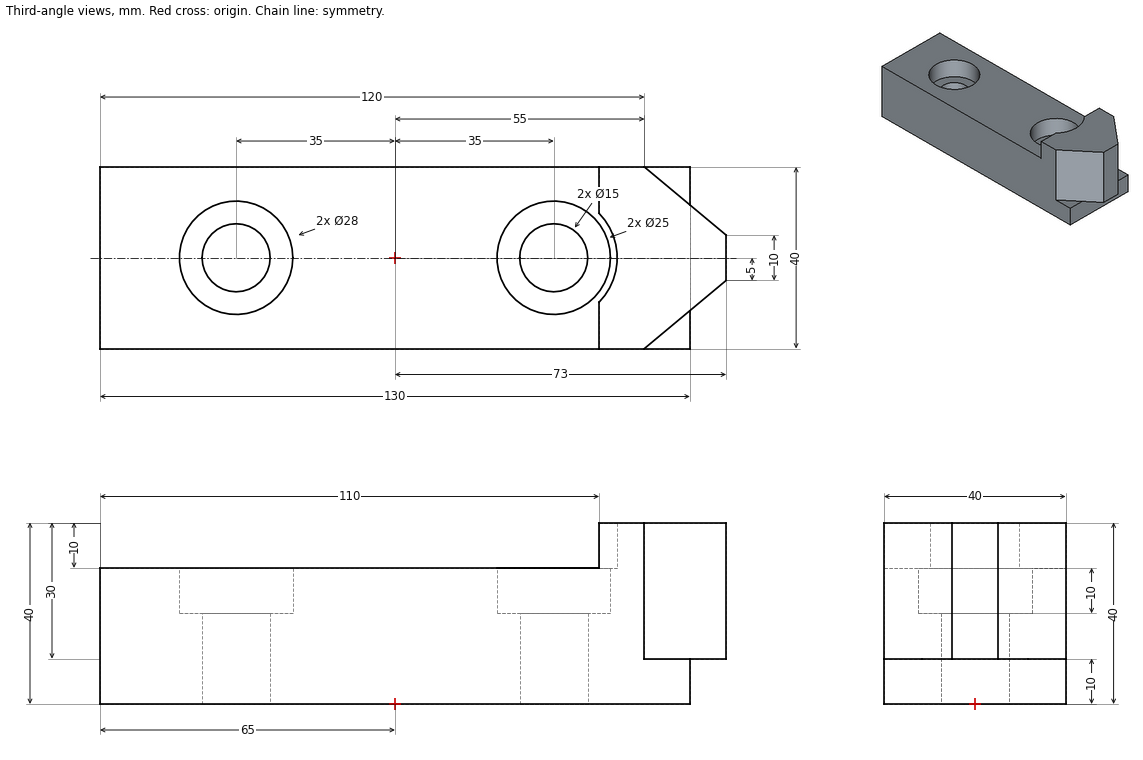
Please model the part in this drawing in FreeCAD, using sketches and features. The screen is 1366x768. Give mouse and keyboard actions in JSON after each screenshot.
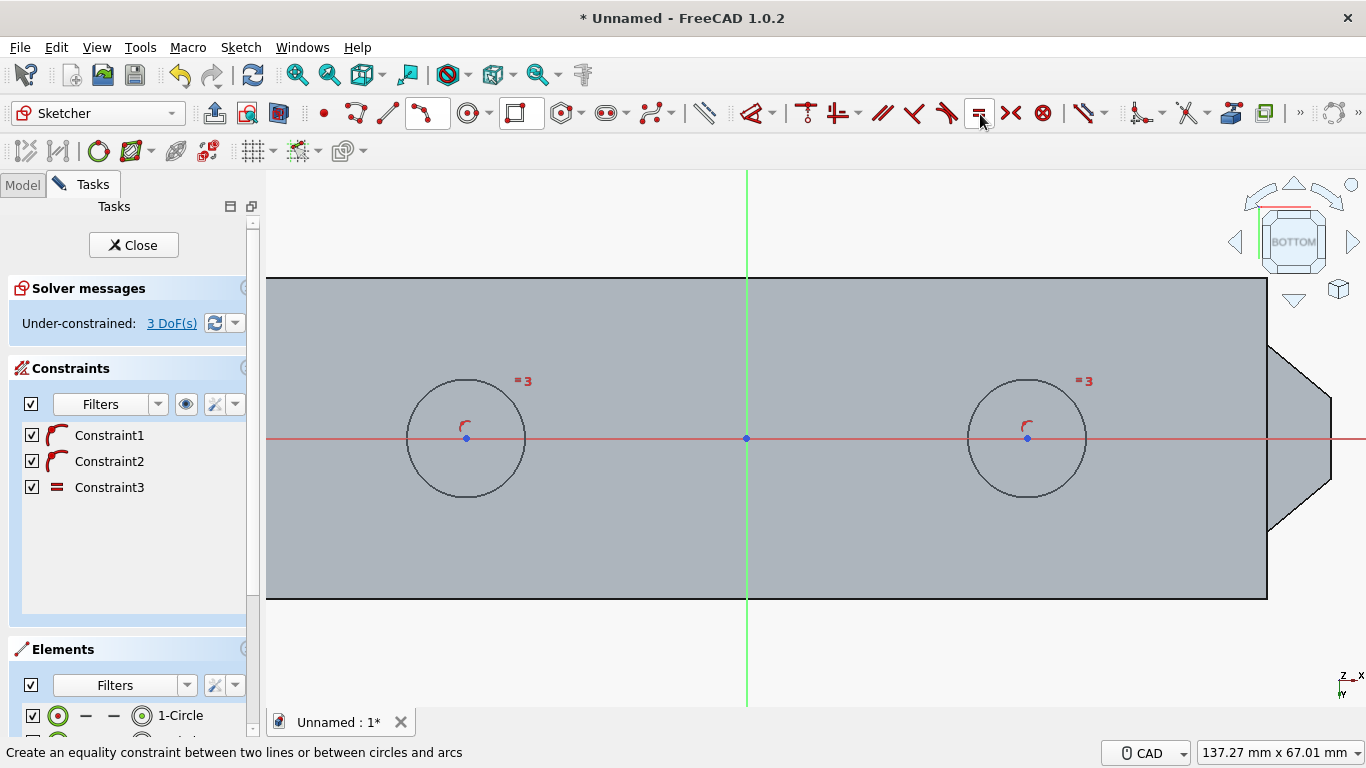
{"action": "left_click", "coordinate": [752, 114]}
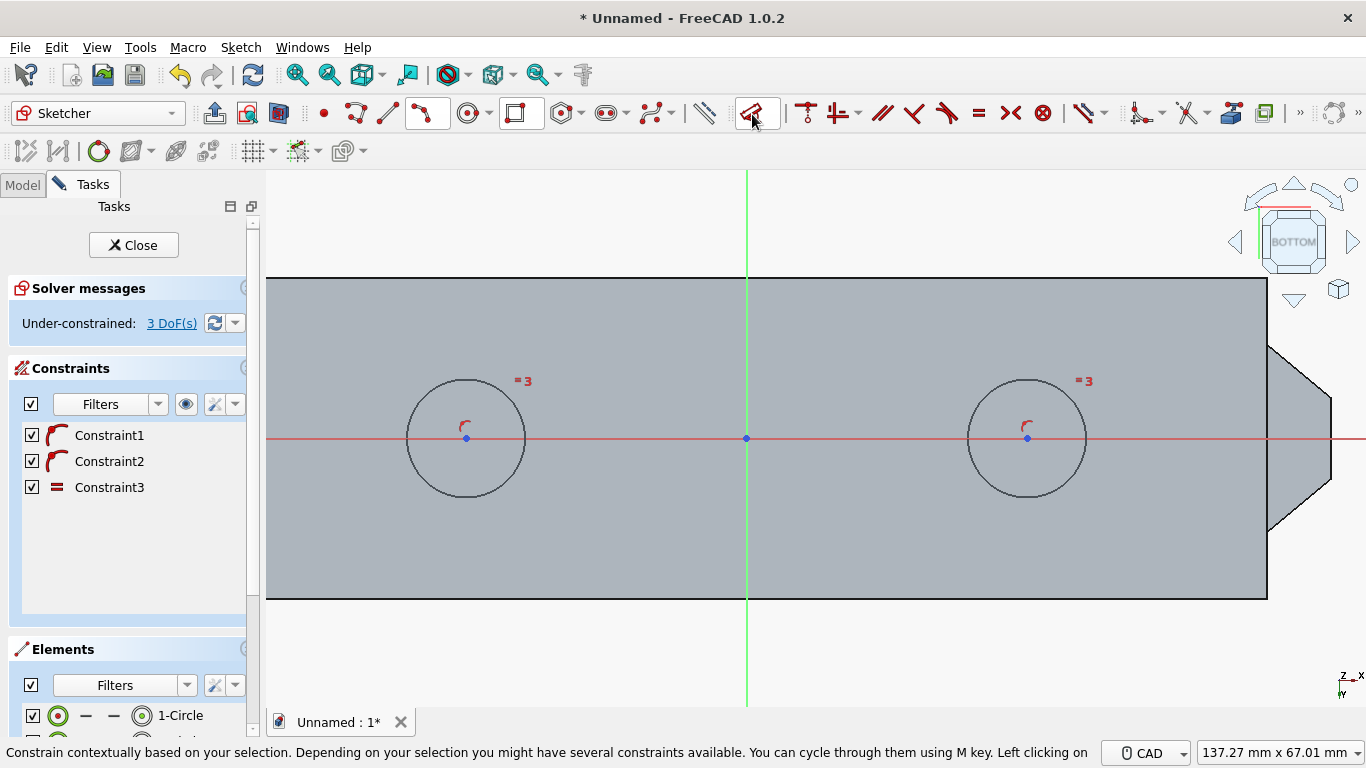
{"action": "left_click", "coordinate": [1069, 397]}
{"action": "left_click", "coordinate": [1092, 375]}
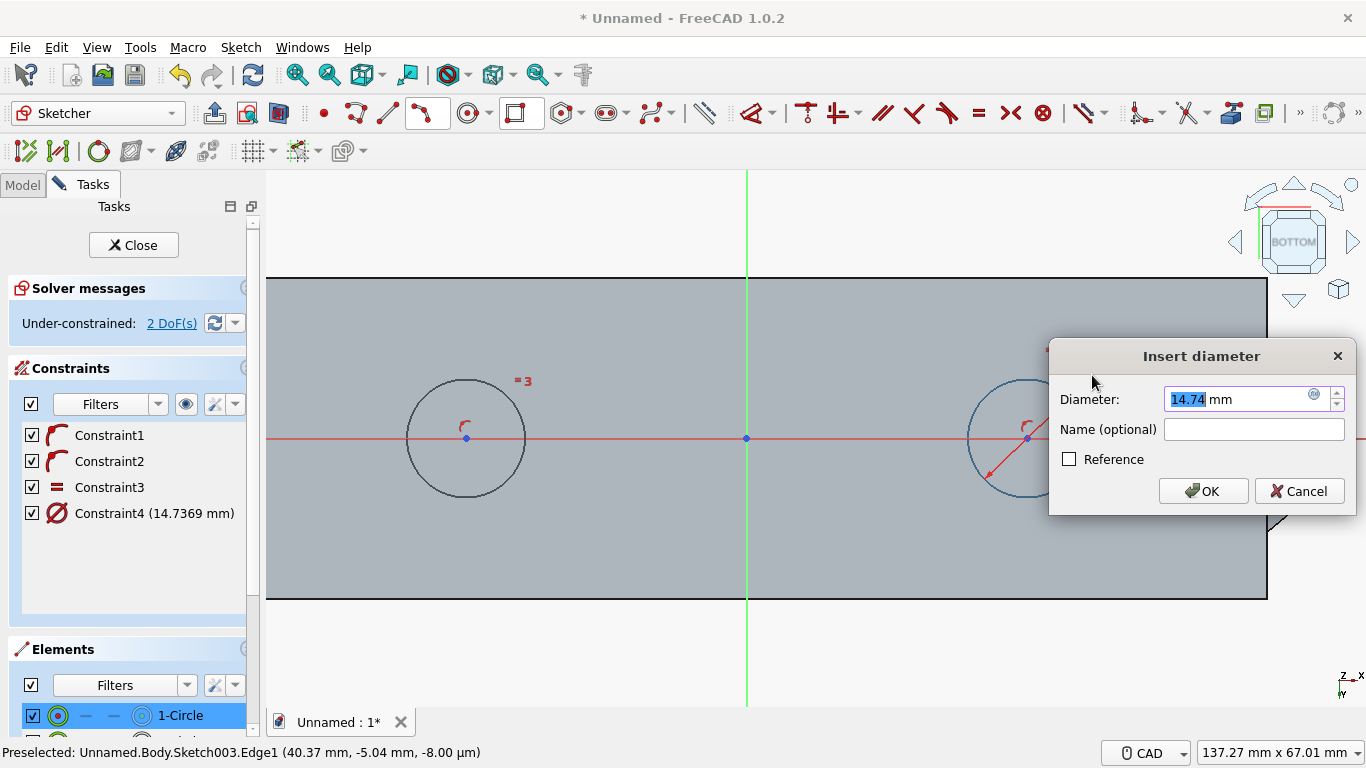
{"action": "type", "text": "15"}
{"action": "key", "text": "Return"}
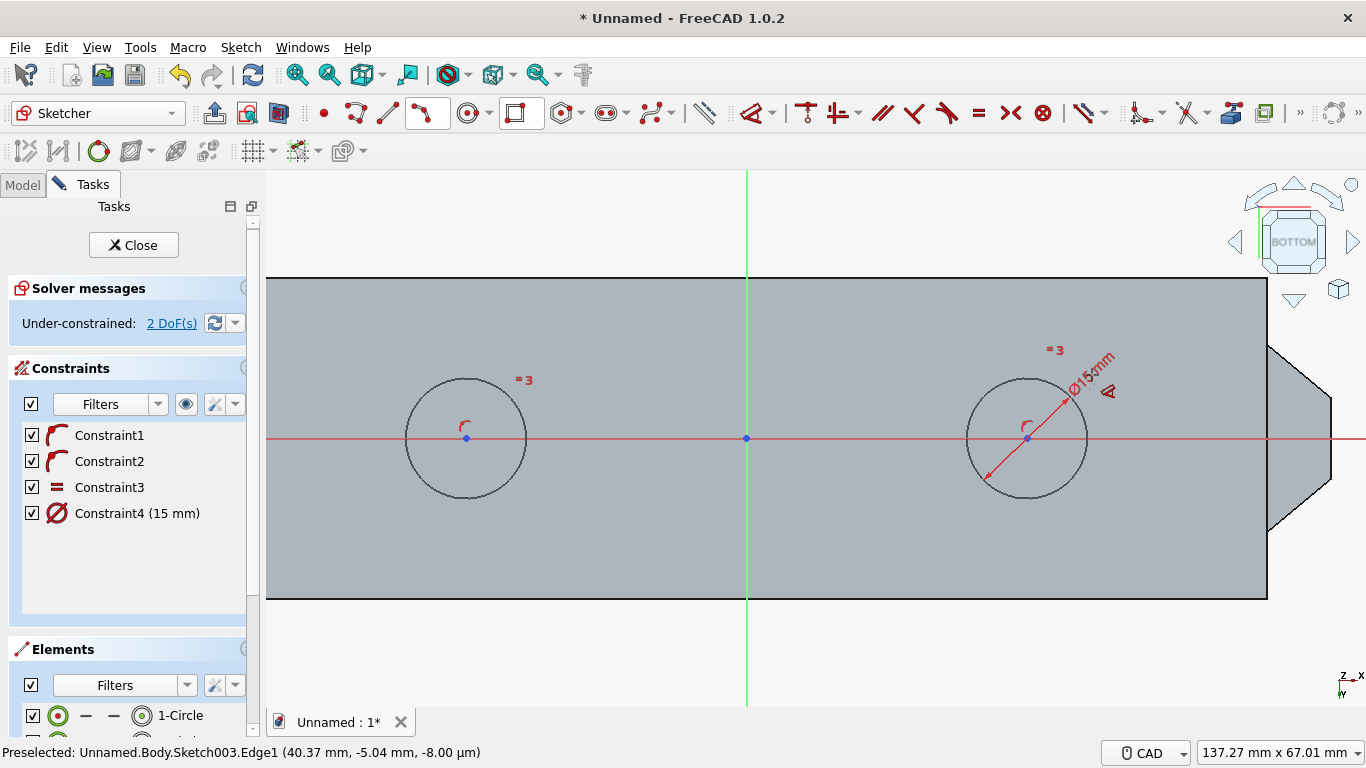
{"action": "left_click", "coordinate": [1027, 438]}
{"action": "left_click", "coordinate": [887, 472]}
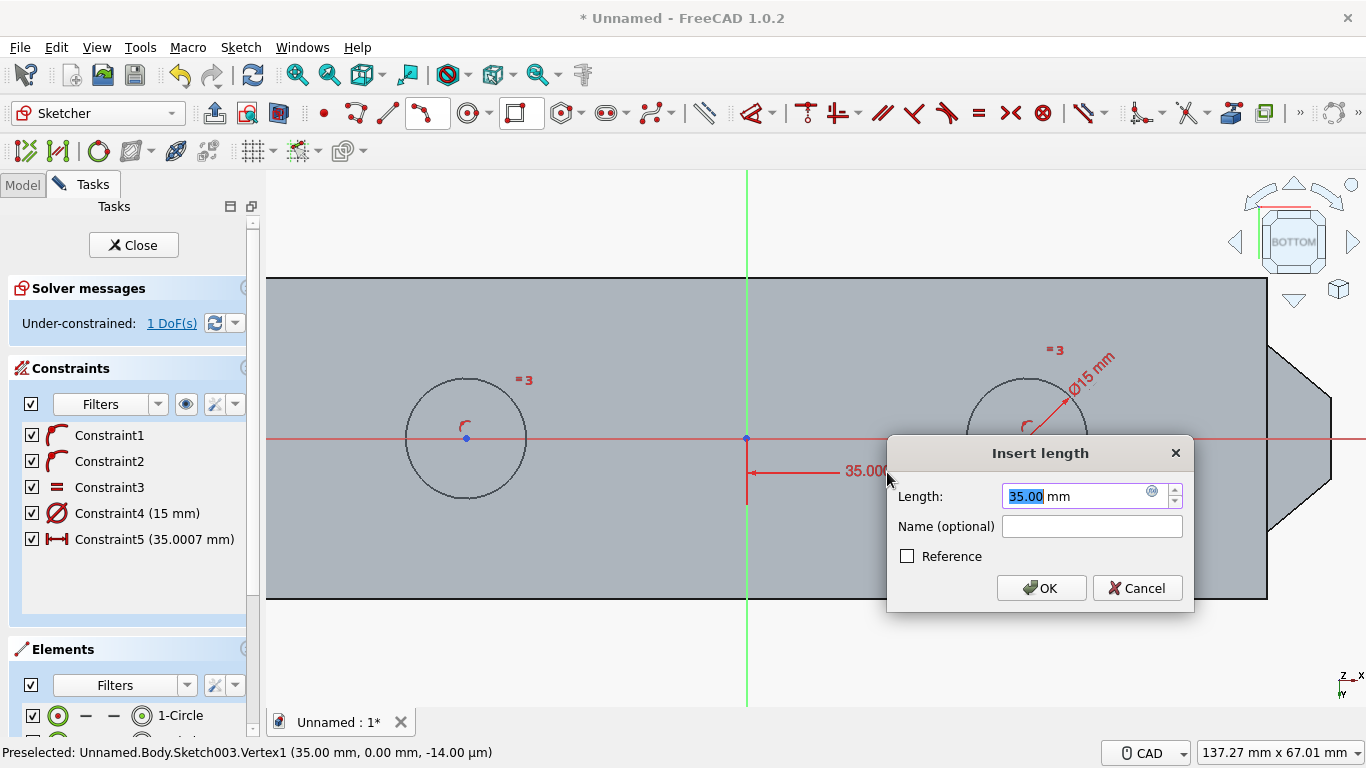
{"action": "type", "text": "35"}
{"action": "key", "text": "Return"}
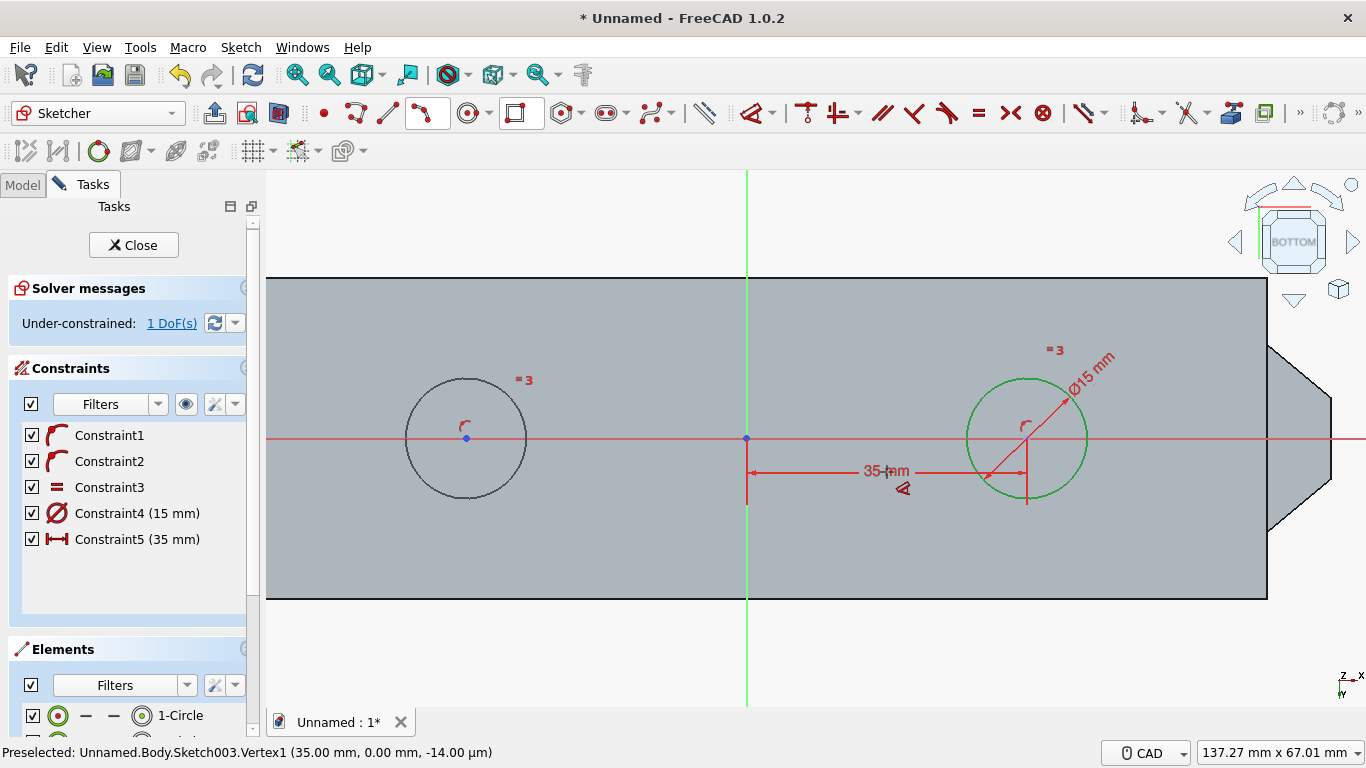
{"action": "left_click", "coordinate": [466, 438]}
{"action": "left_click", "coordinate": [606, 472]}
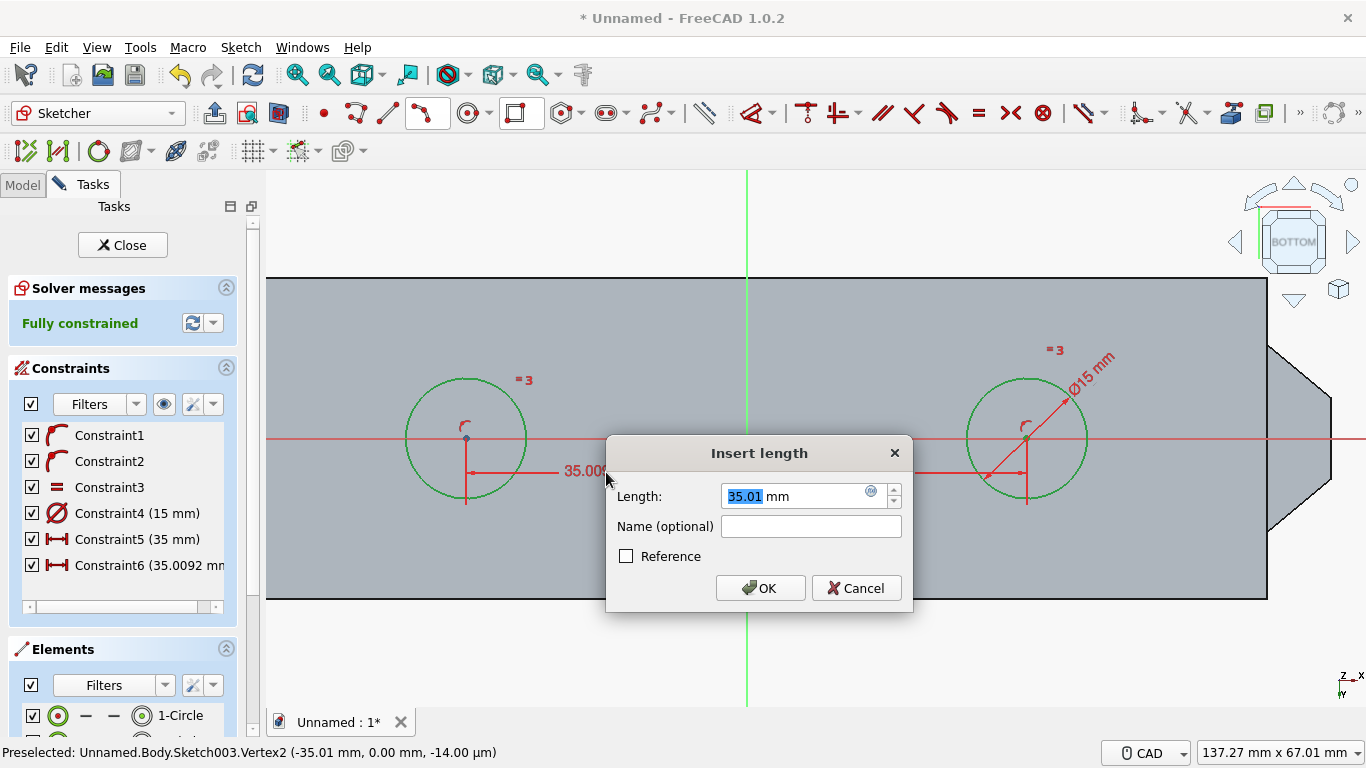
{"action": "type", "text": "35"}
{"action": "key", "text": "Return"}
{"action": "key", "text": "Escape"}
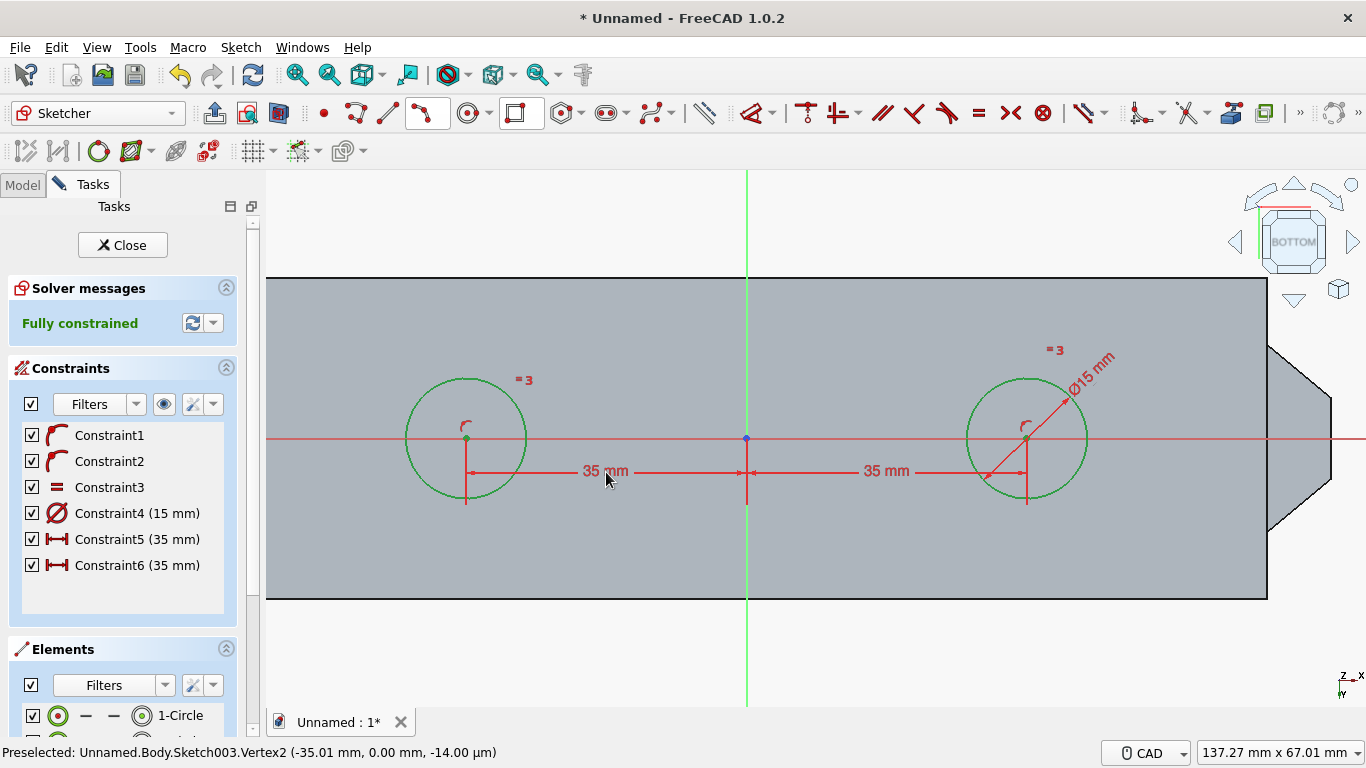
{"action": "left_click", "coordinate": [123, 245]}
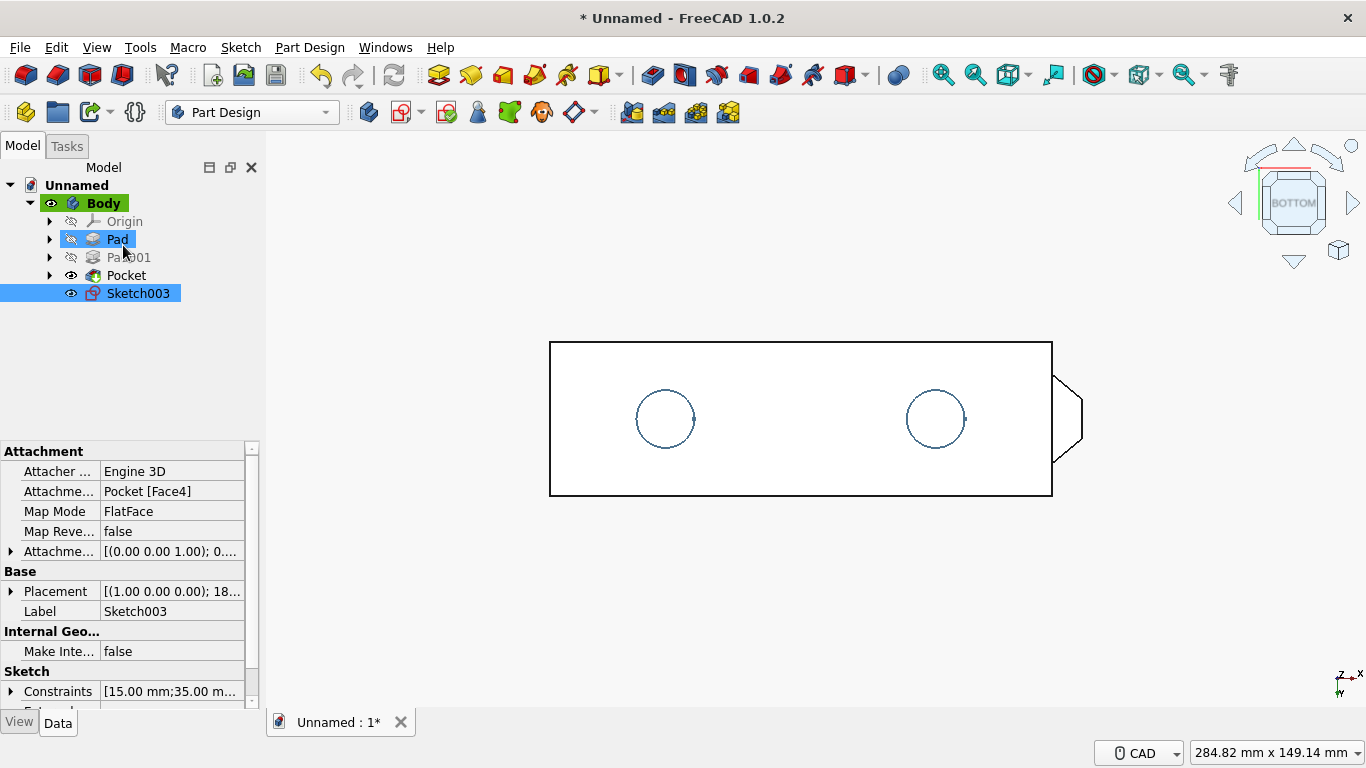
{"action": "left_click", "coordinate": [654, 76]}